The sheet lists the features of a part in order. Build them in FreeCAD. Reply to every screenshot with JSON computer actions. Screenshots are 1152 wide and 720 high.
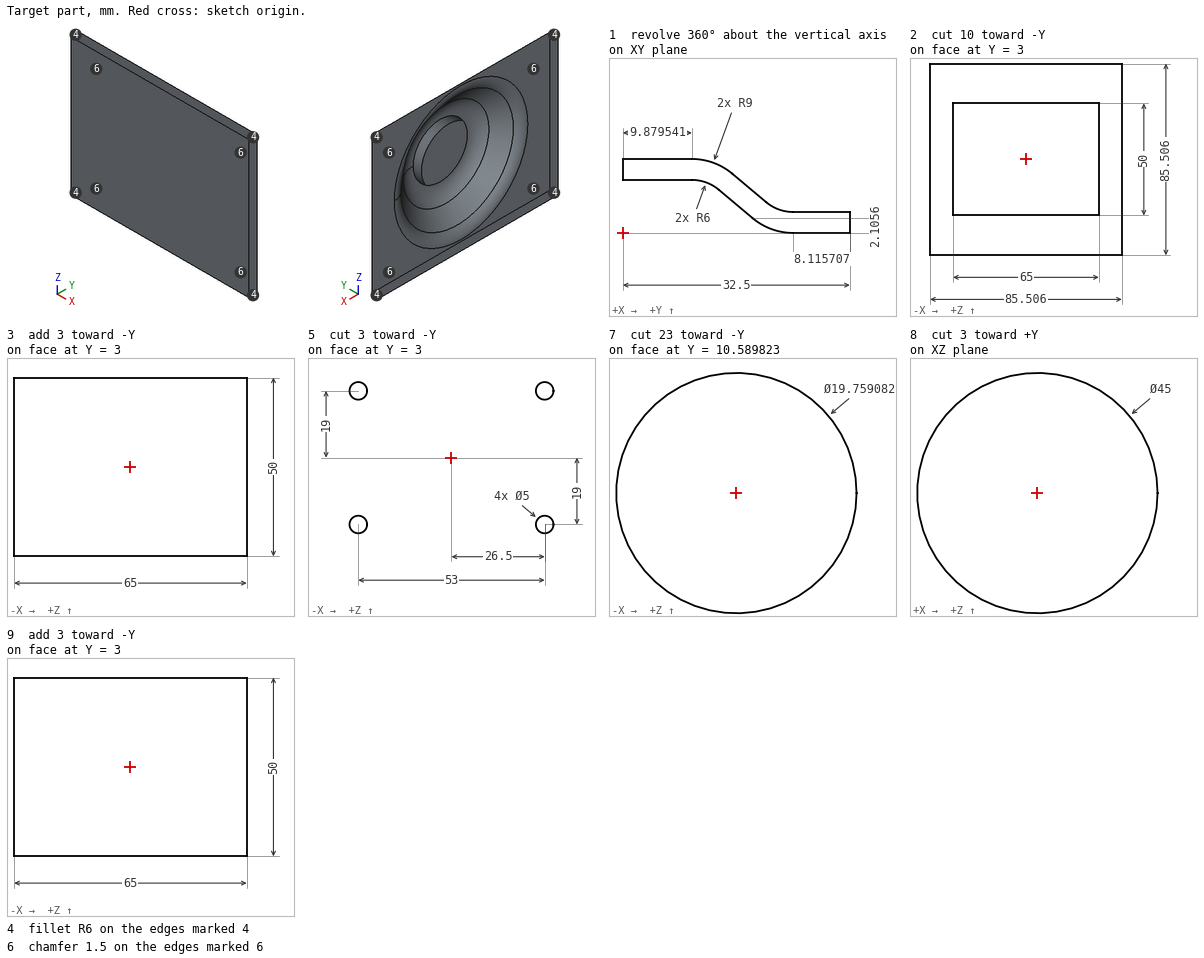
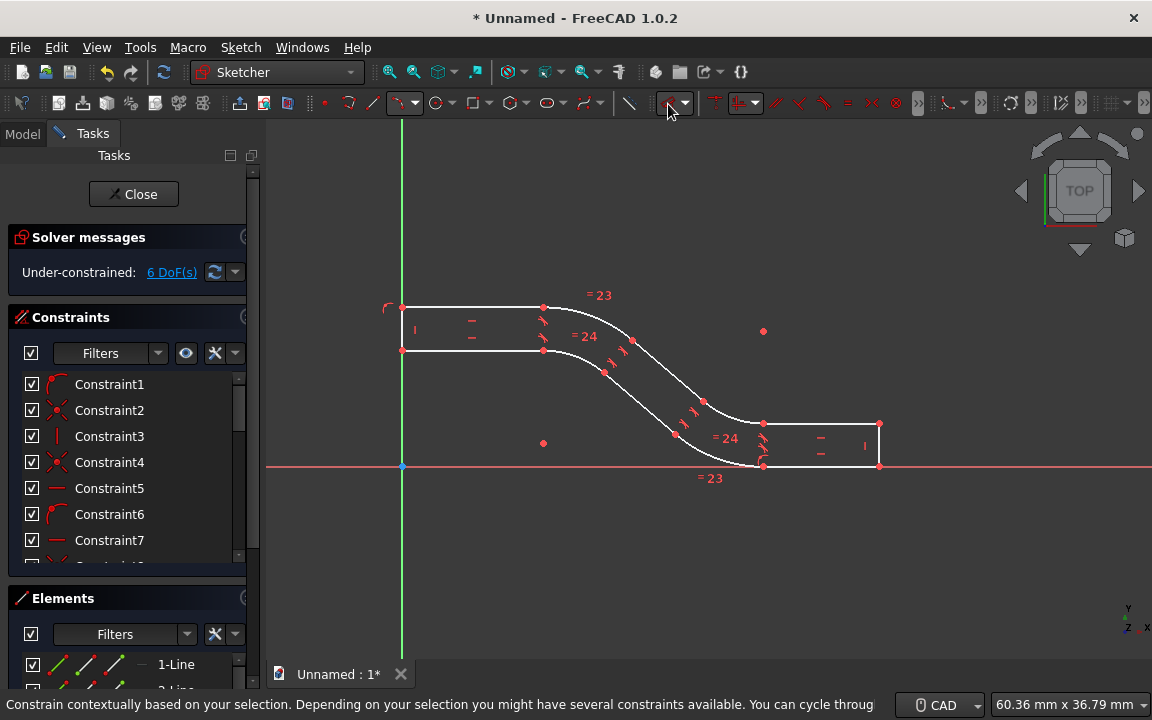
{"action": "left_click", "coordinate": [699, 451]}
{"action": "left_click", "coordinate": [623, 423]}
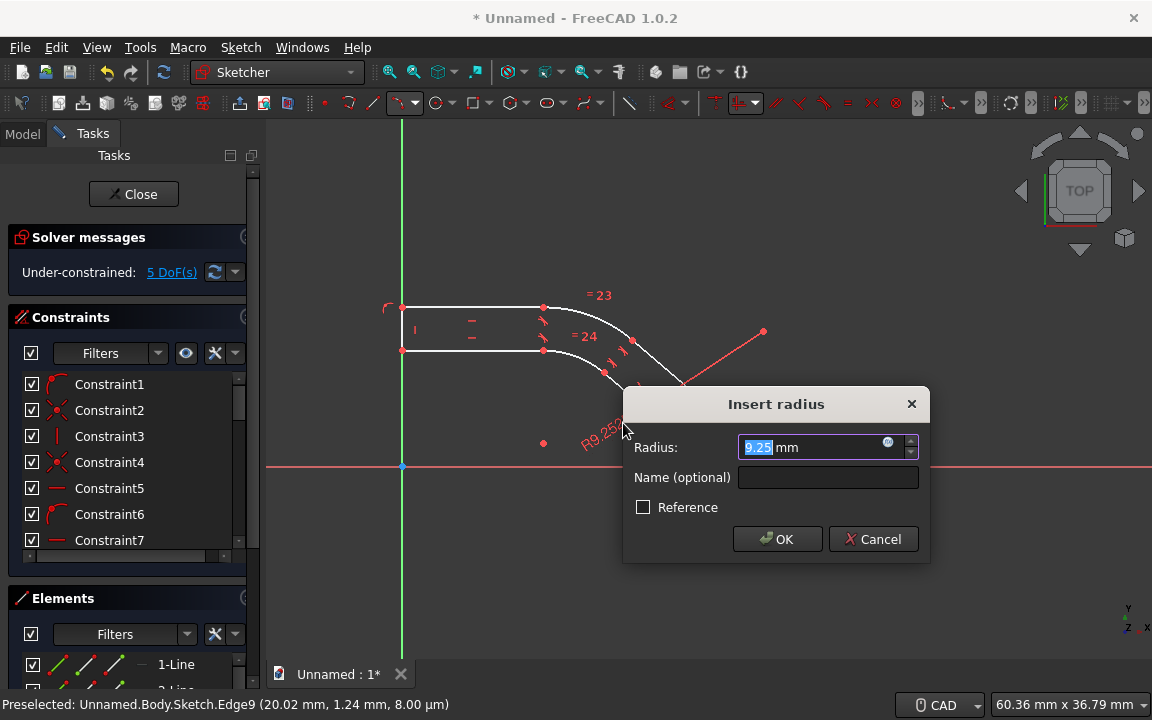
{"action": "type", "text": "9"}
{"action": "key", "text": "Return"}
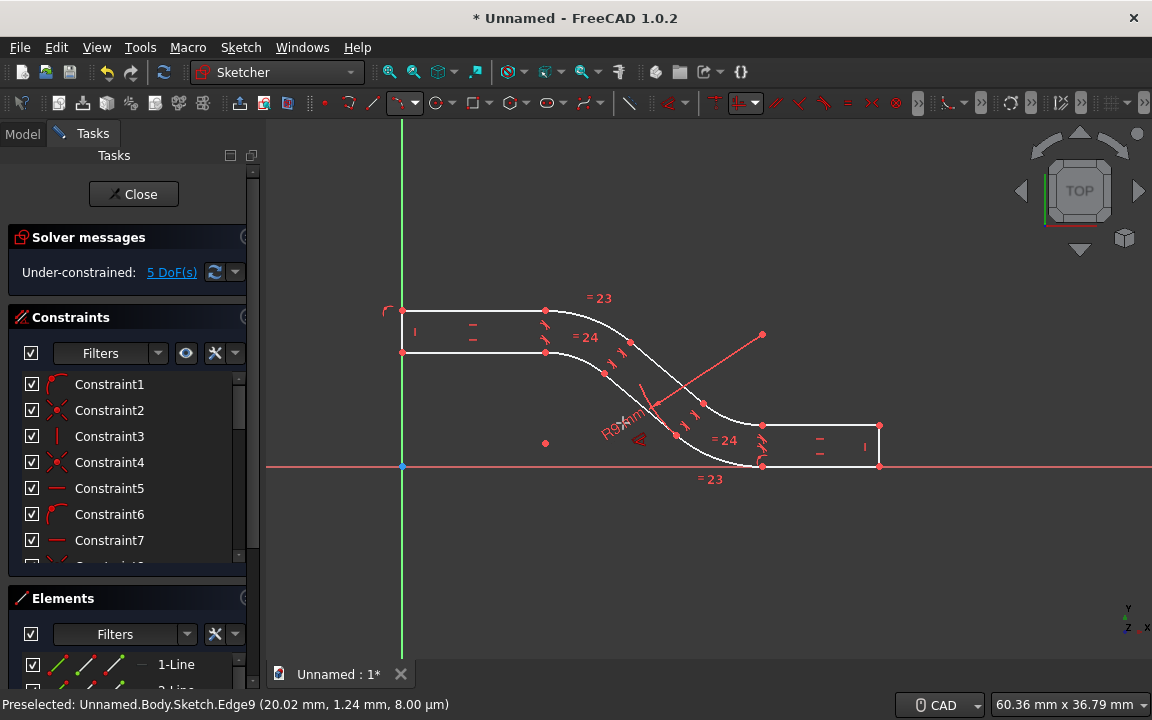
{"action": "left_click", "coordinate": [719, 415]}
{"action": "left_click", "coordinate": [659, 402]}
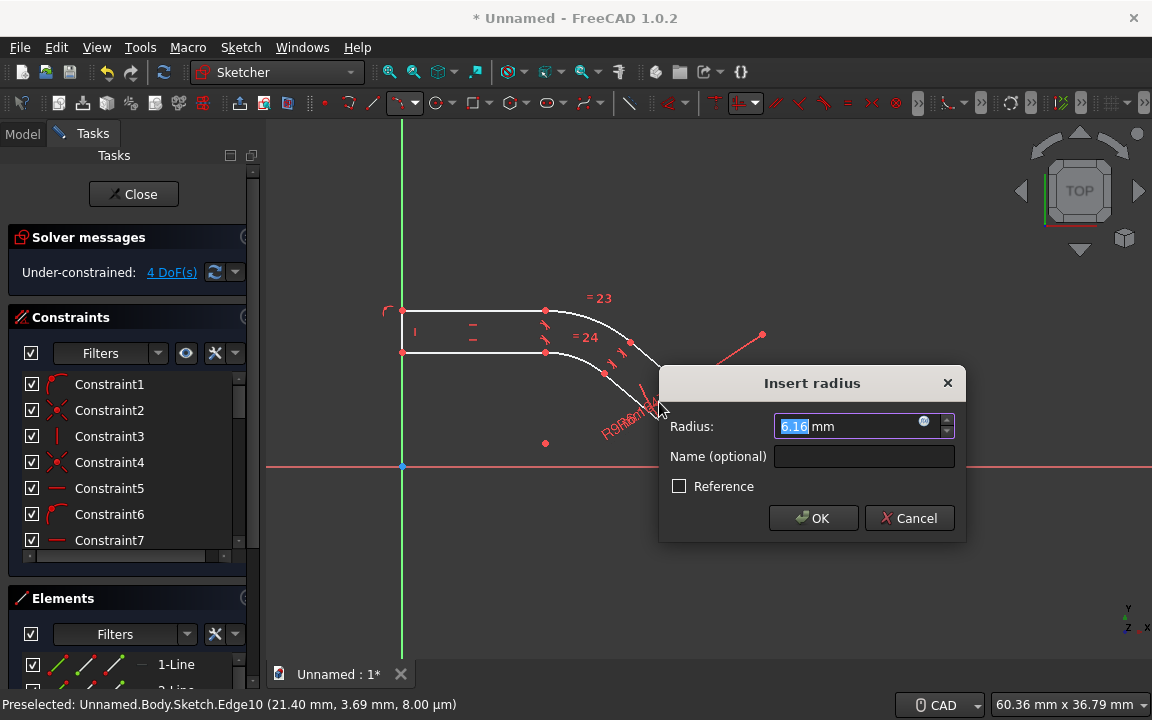
{"action": "type", "text": "6"}
{"action": "key", "text": "Return"}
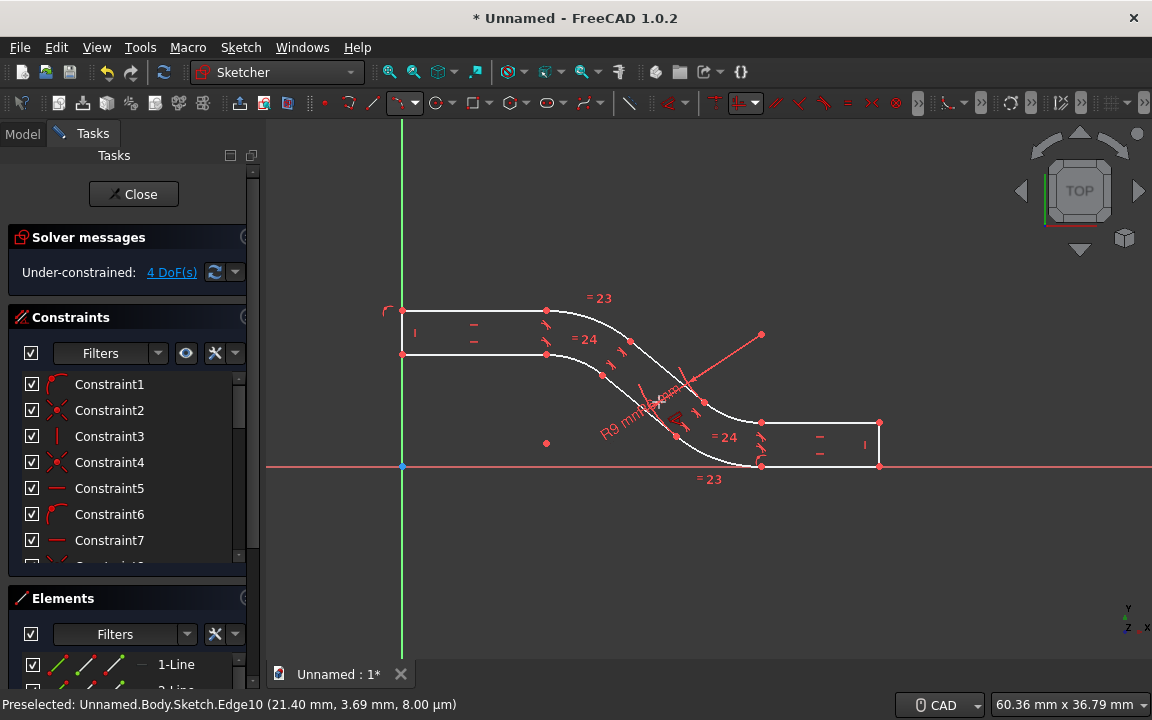
{"action": "left_click", "coordinate": [879, 467]}
{"action": "left_click", "coordinate": [641, 501]}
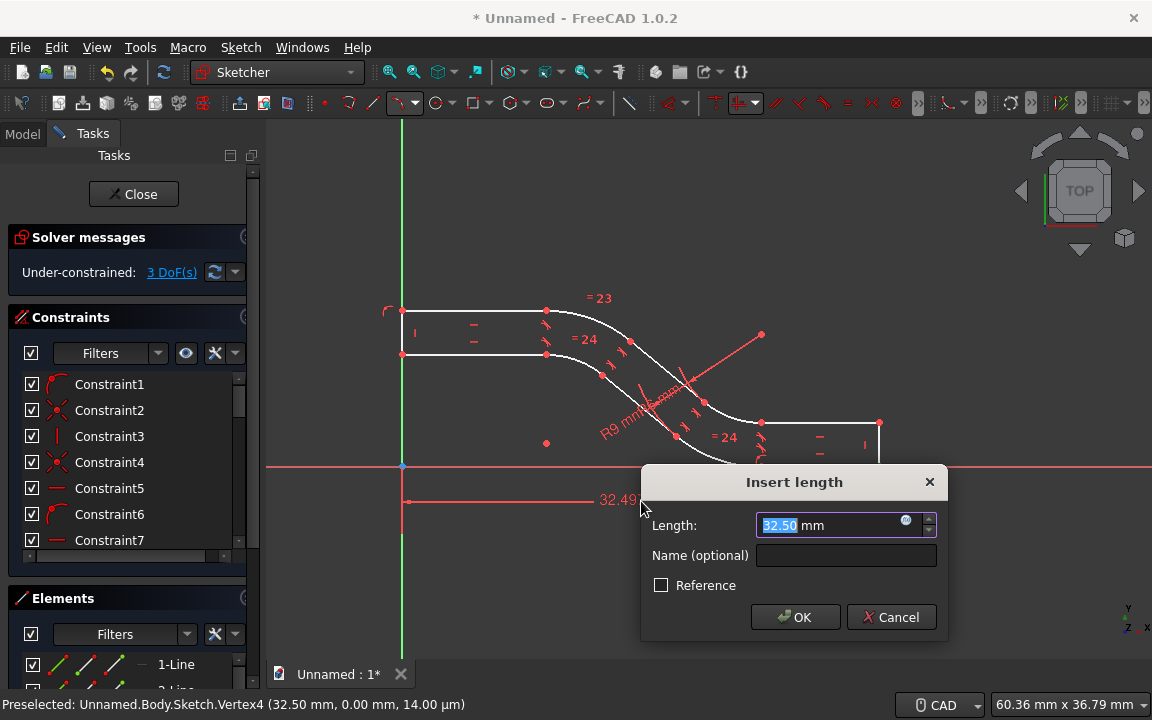
{"action": "type", "text": "32.5"}
{"action": "key", "text": "Return"}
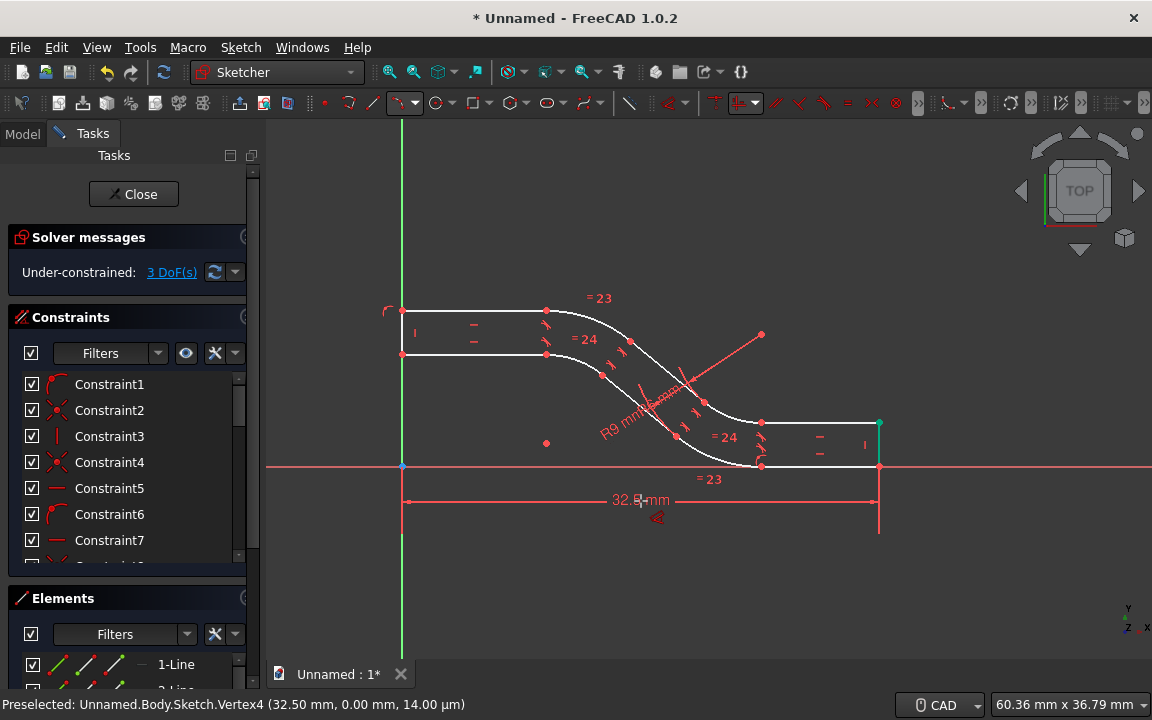
{"action": "scroll", "coordinate": [677, 436], "scroll_direction": "up", "scroll_amount": 2}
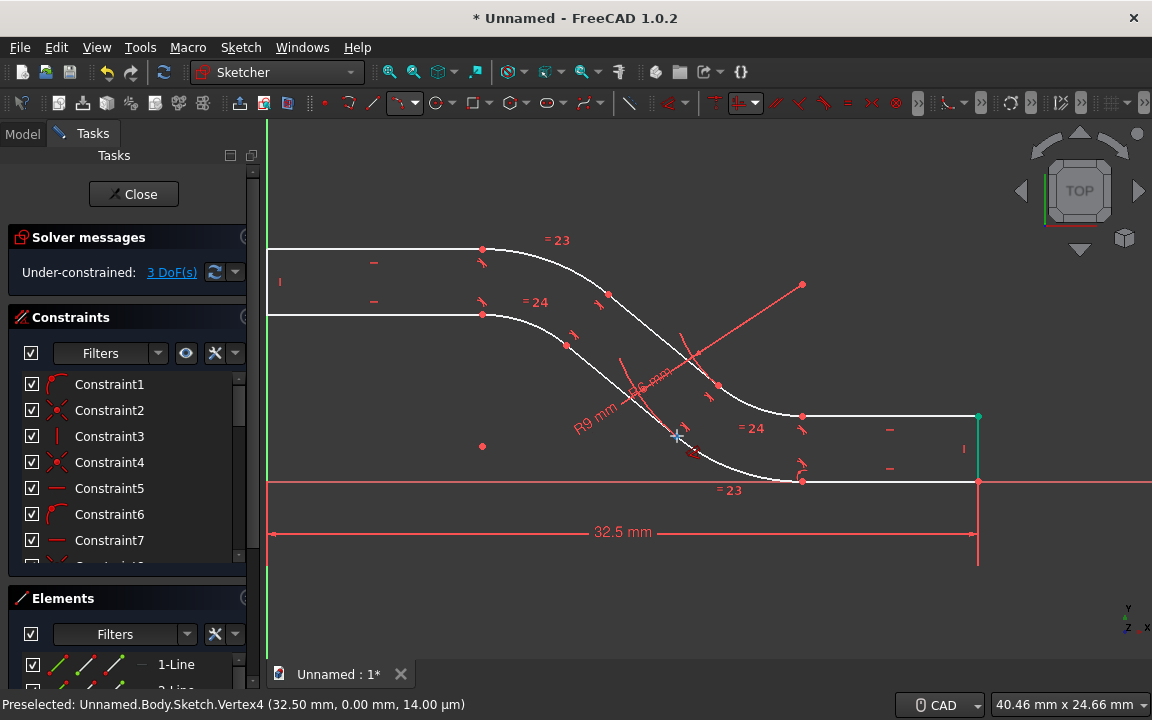
{"action": "left_click", "coordinate": [677, 436]}
{"action": "left_click", "coordinate": [711, 443]}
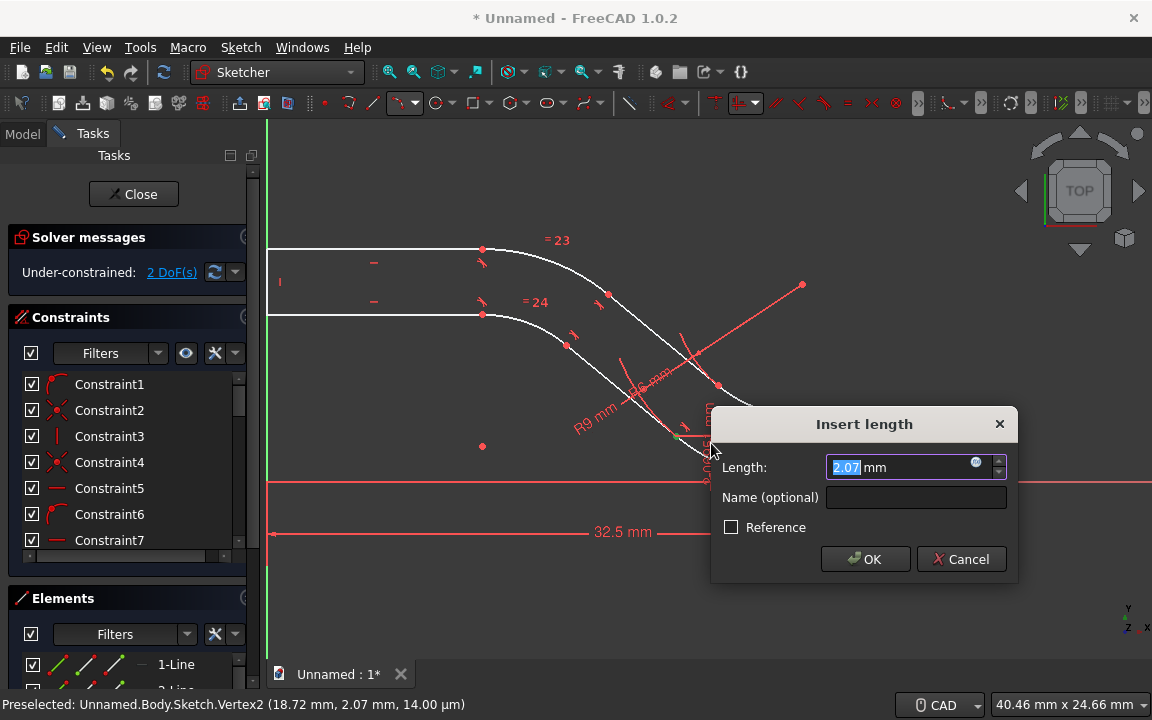
{"action": "type", "text": "2.1056"}
{"action": "key", "text": "Return"}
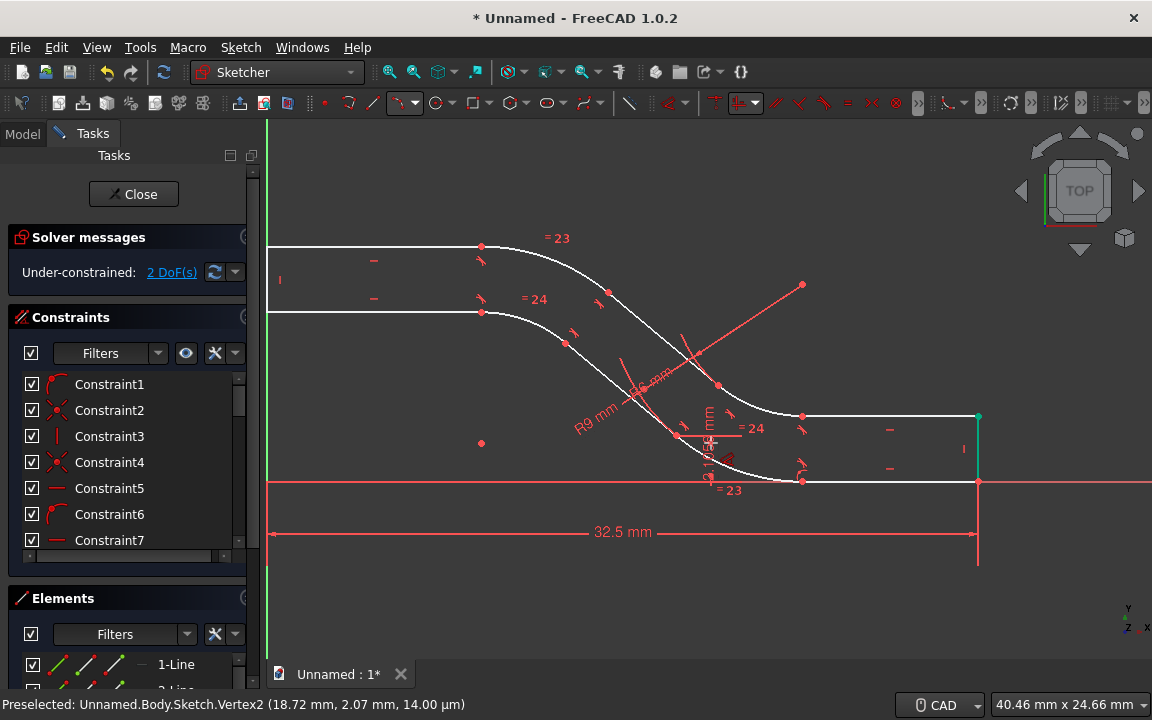
{"action": "left_click", "coordinate": [856, 482]}
{"action": "left_click", "coordinate": [891, 516]}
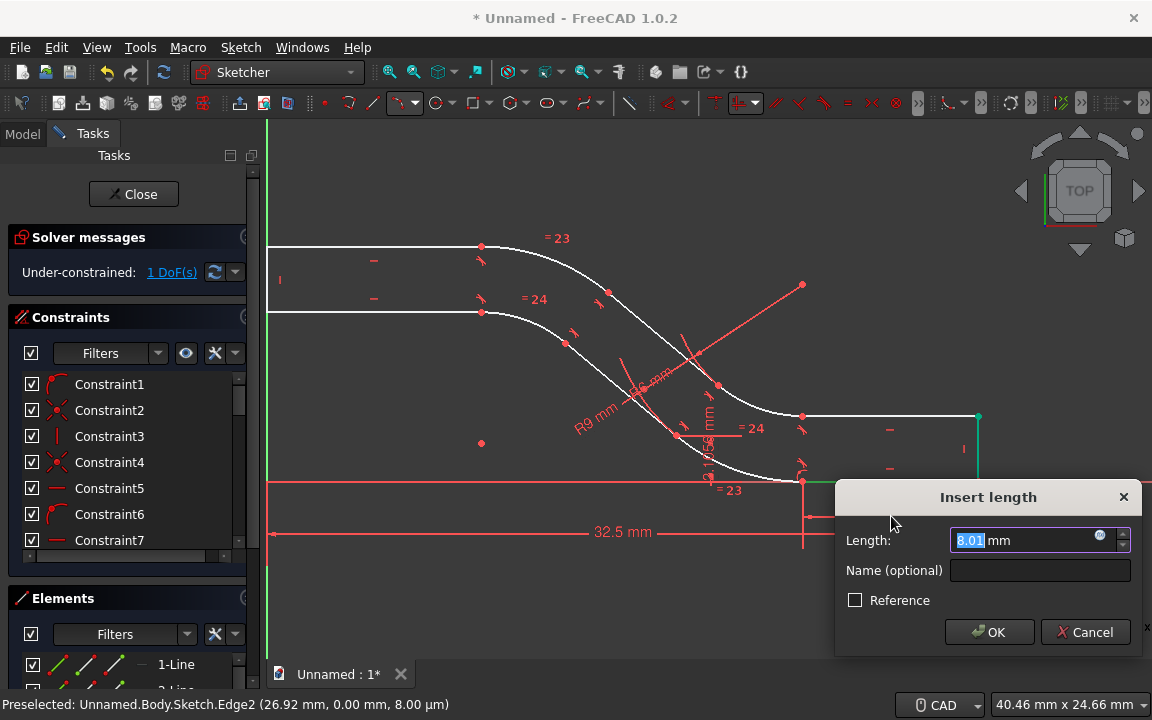
{"action": "type", "text": "8.115707"}
{"action": "key", "text": "Return"}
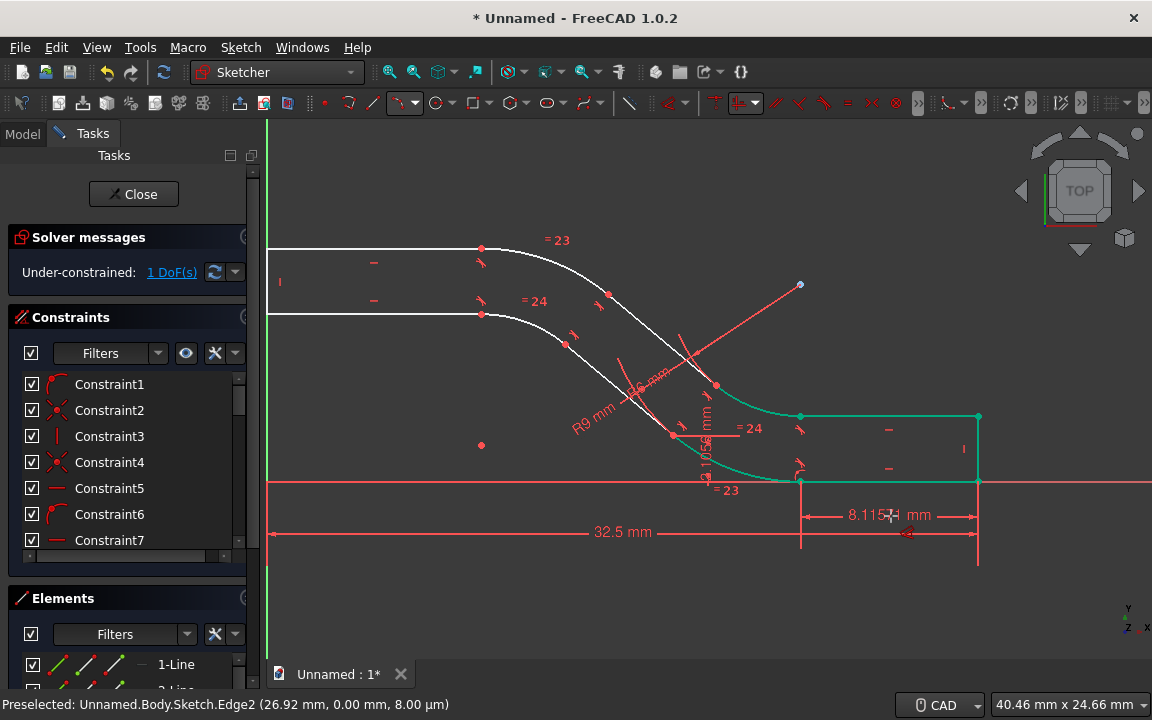
{"action": "left_click", "coordinate": [417, 249]}
{"action": "left_click", "coordinate": [388, 215]}